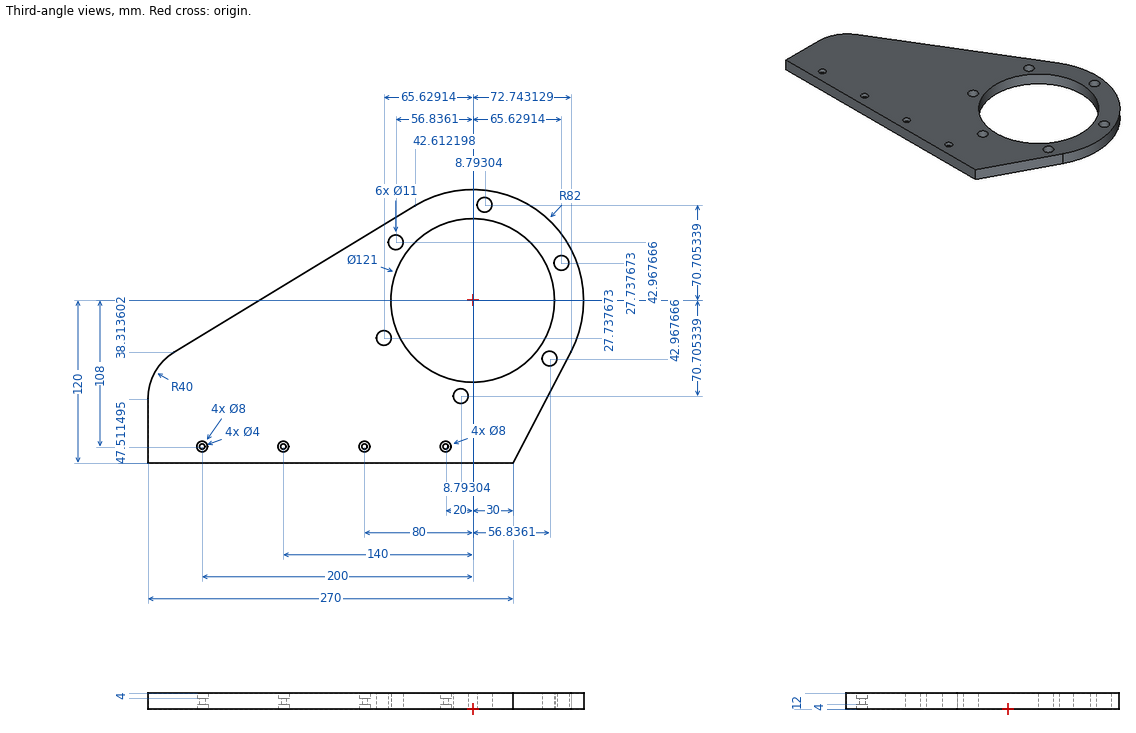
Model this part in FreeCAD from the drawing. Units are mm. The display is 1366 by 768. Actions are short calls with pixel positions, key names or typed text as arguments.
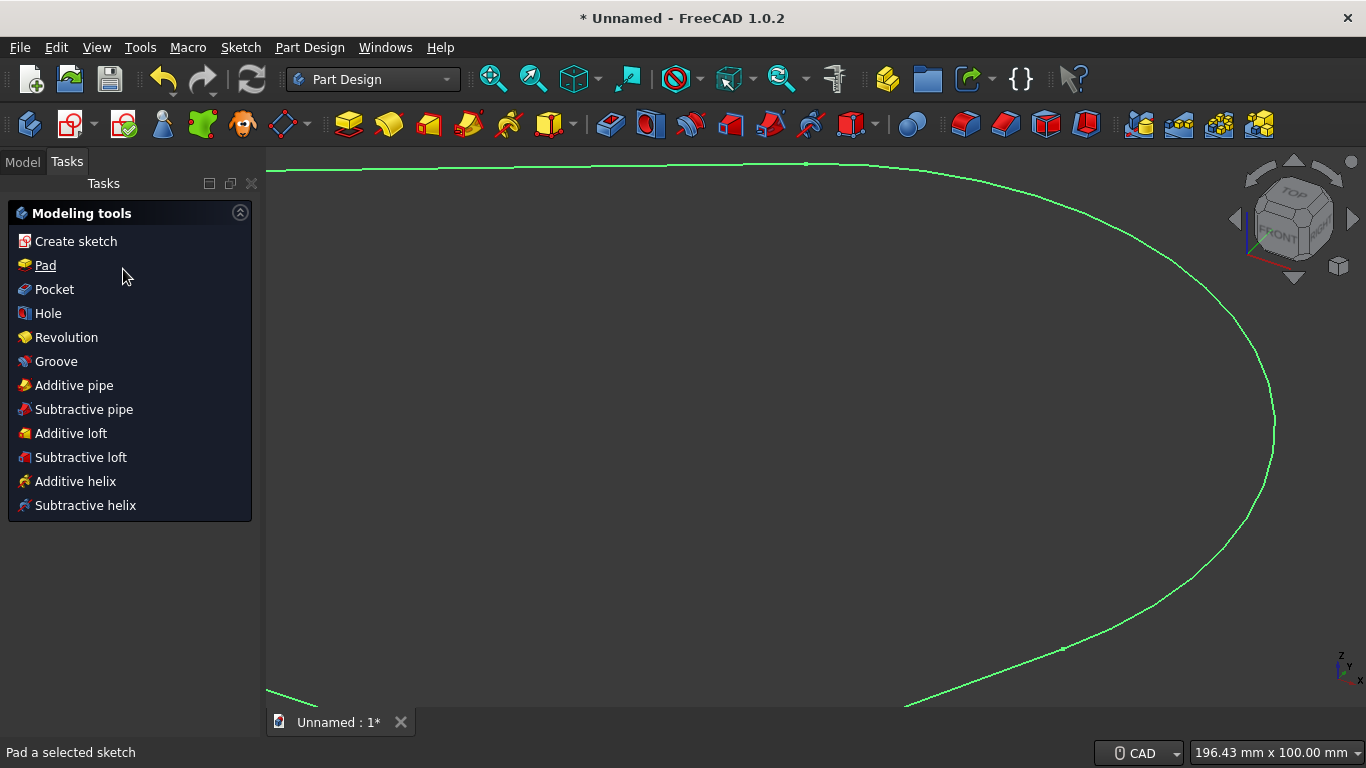
click(350, 124)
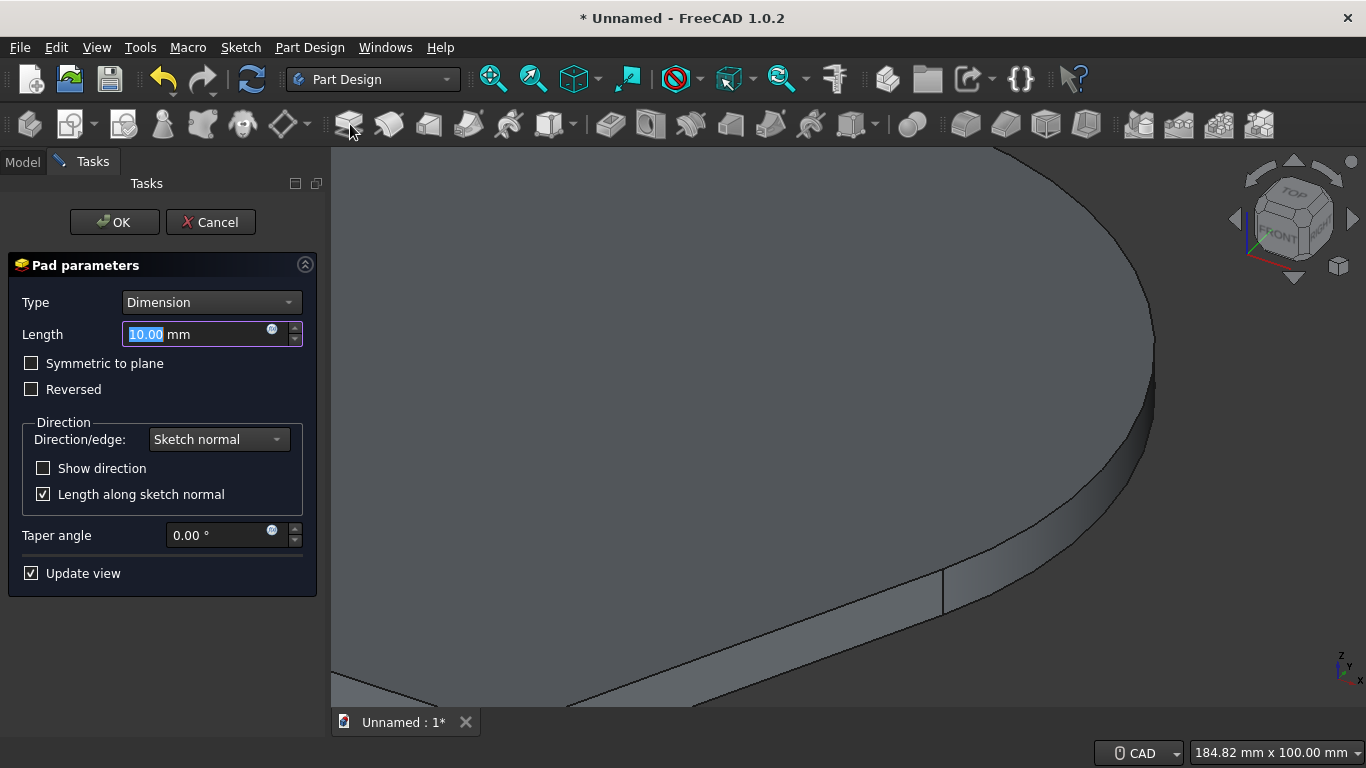
text(12)
key(Tab)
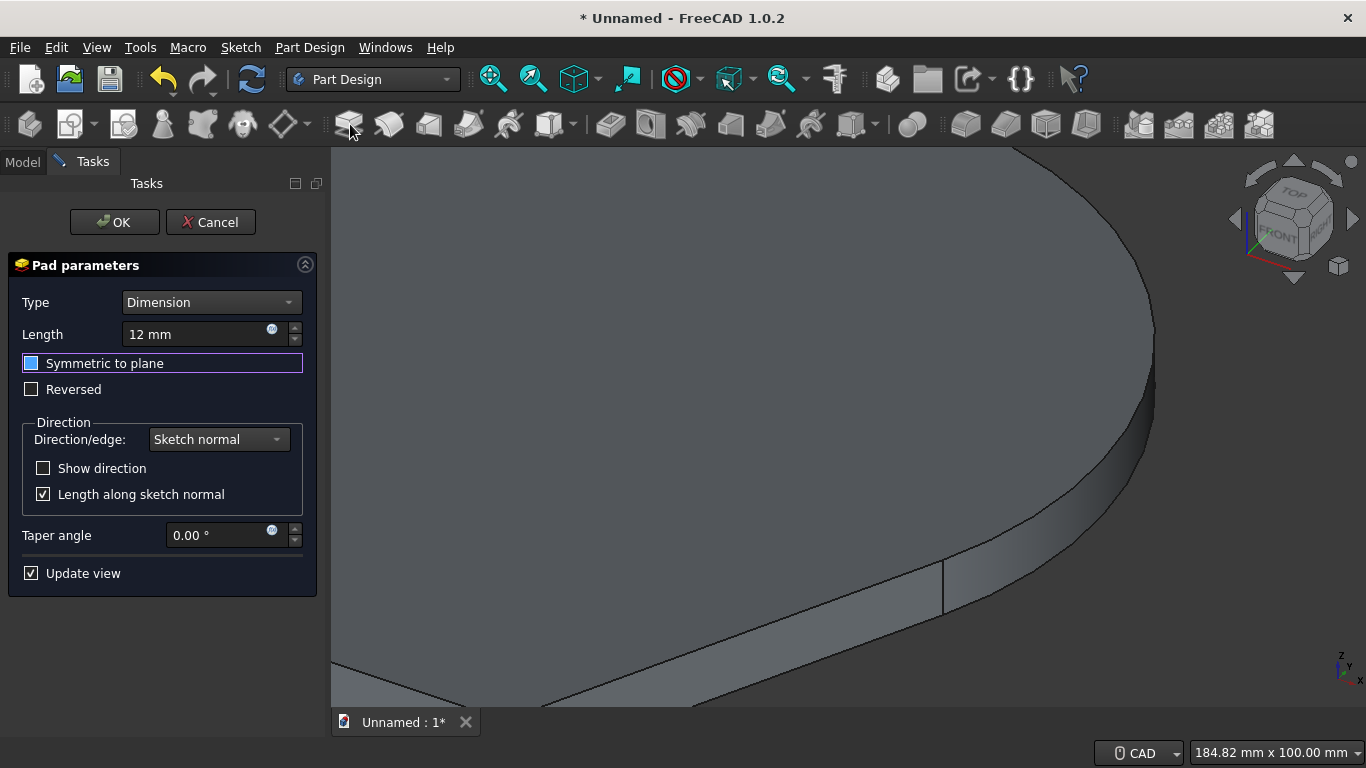
click(115, 222)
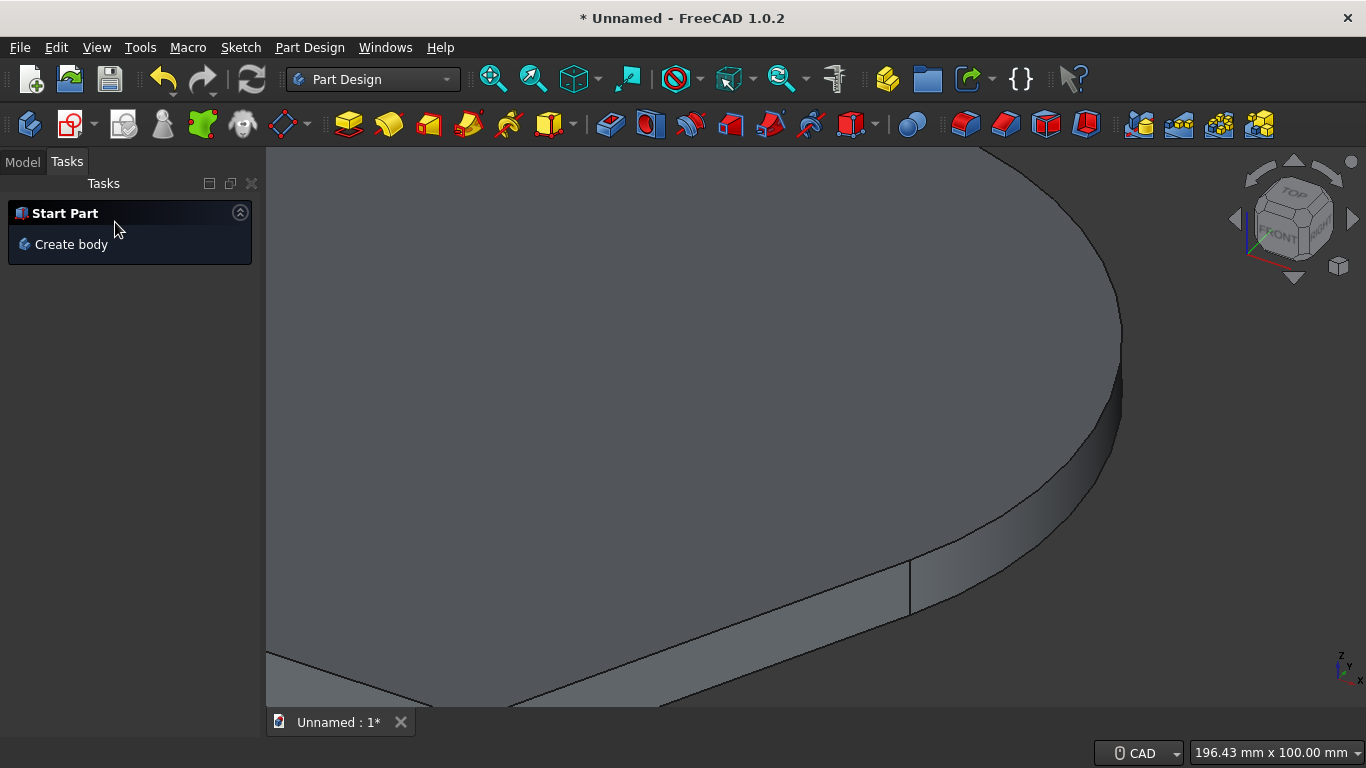
click(494, 80)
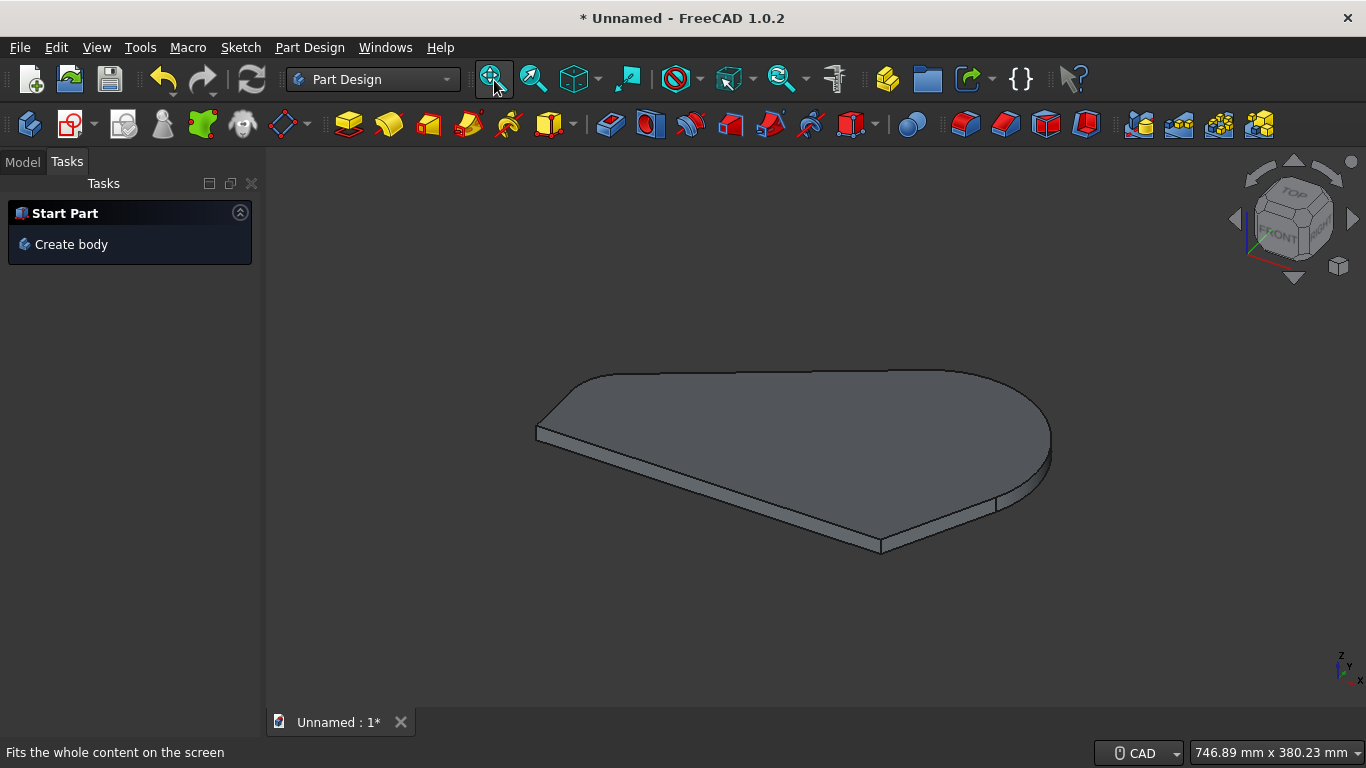
key(5)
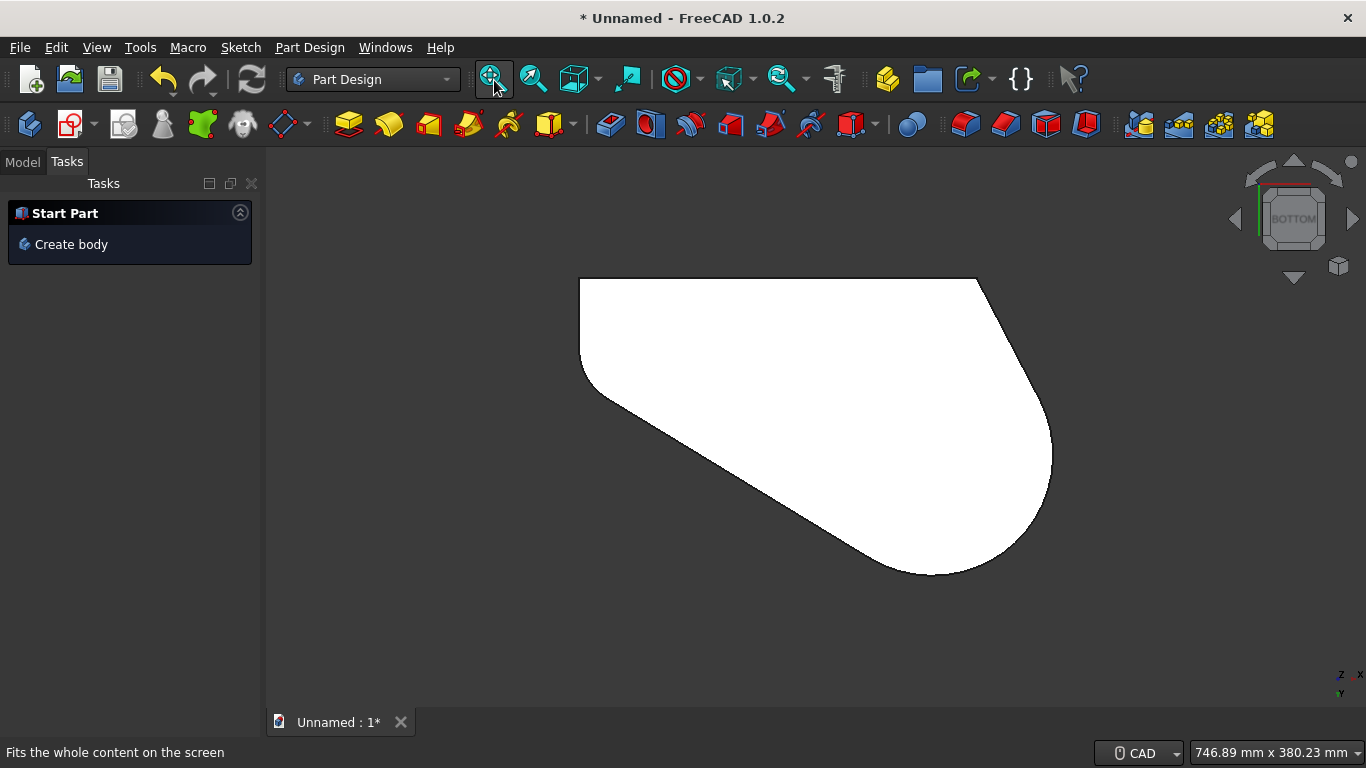
click(884, 426)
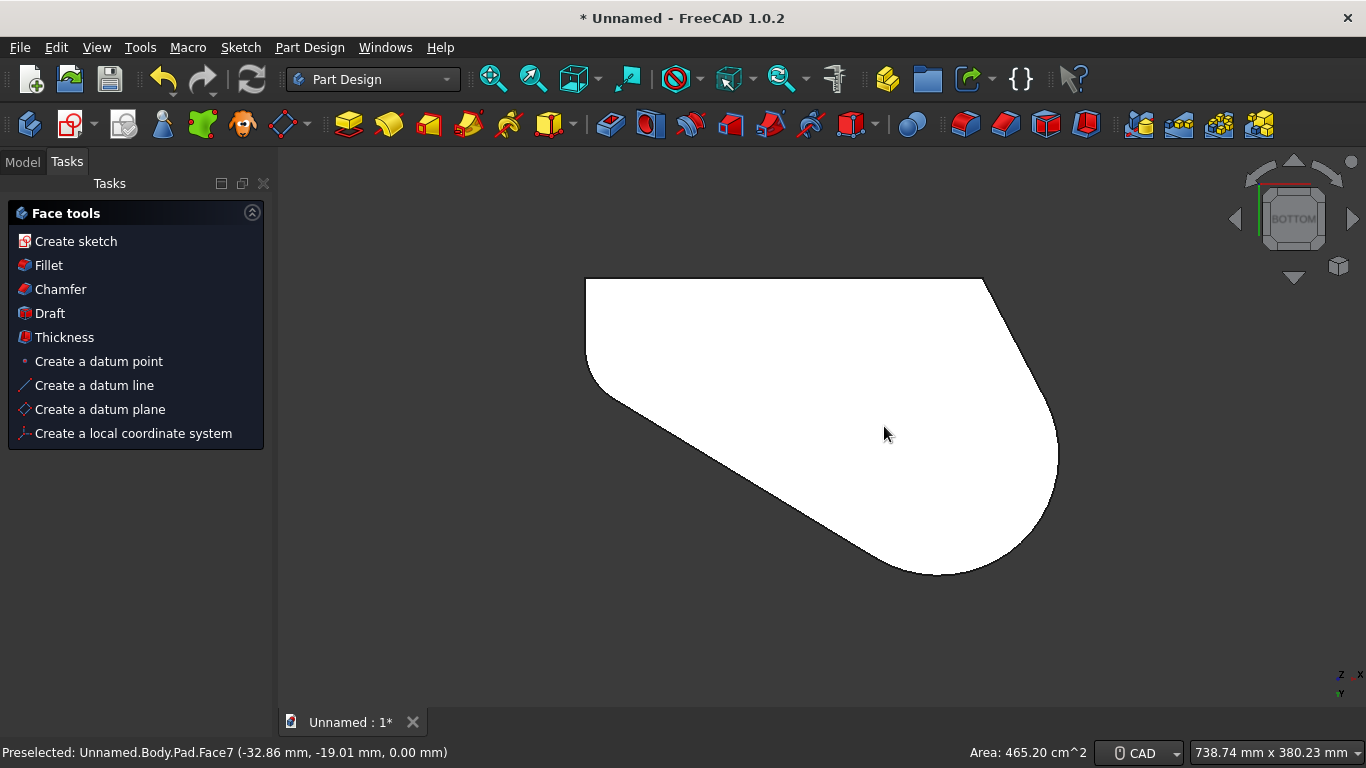
click(70, 124)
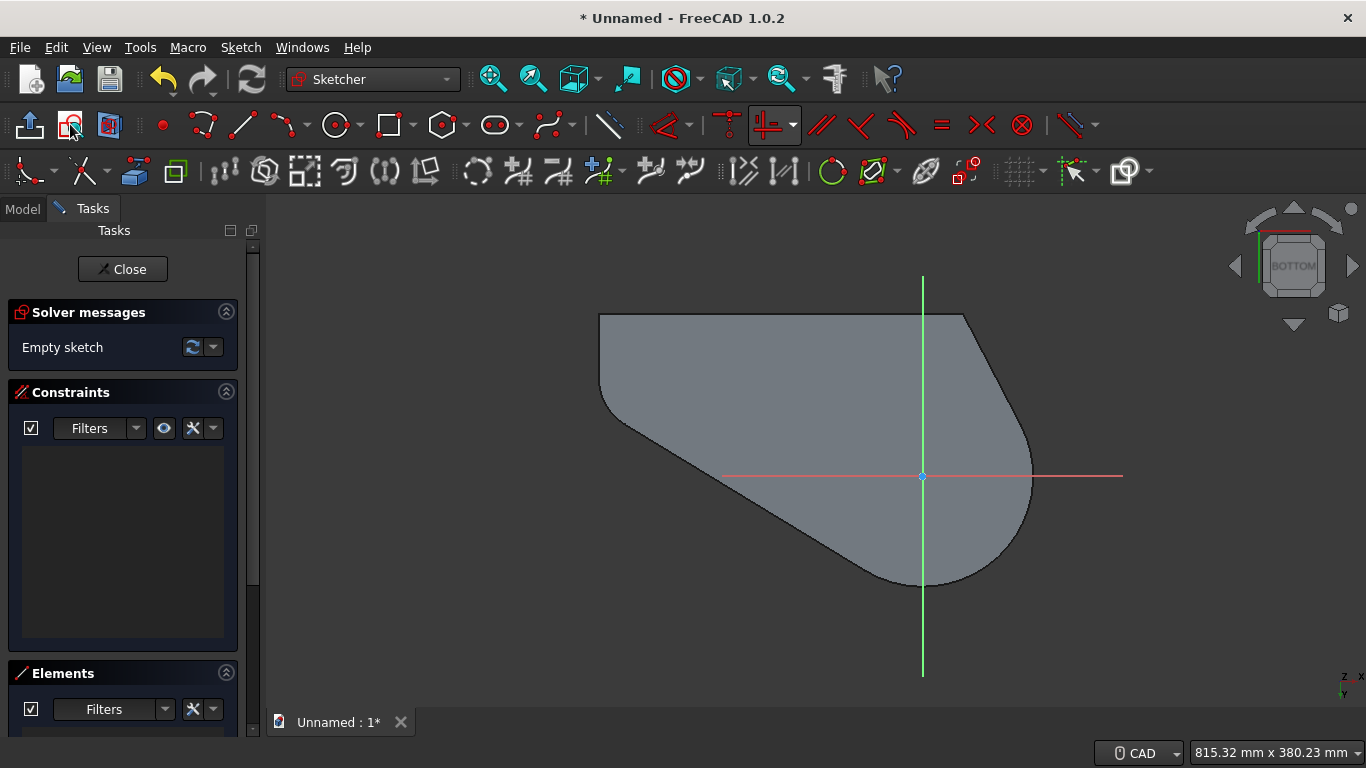
scroll(1136, 507, up, 3)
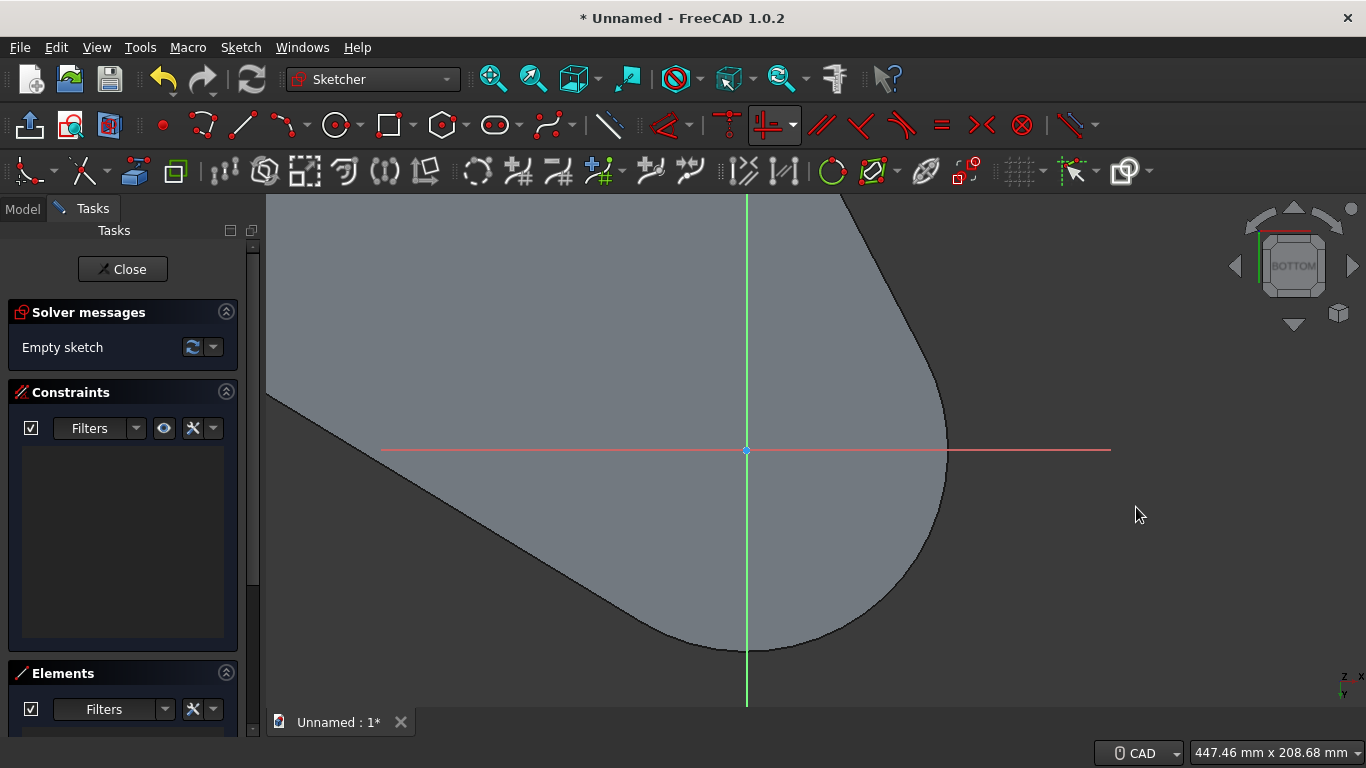
click(336, 126)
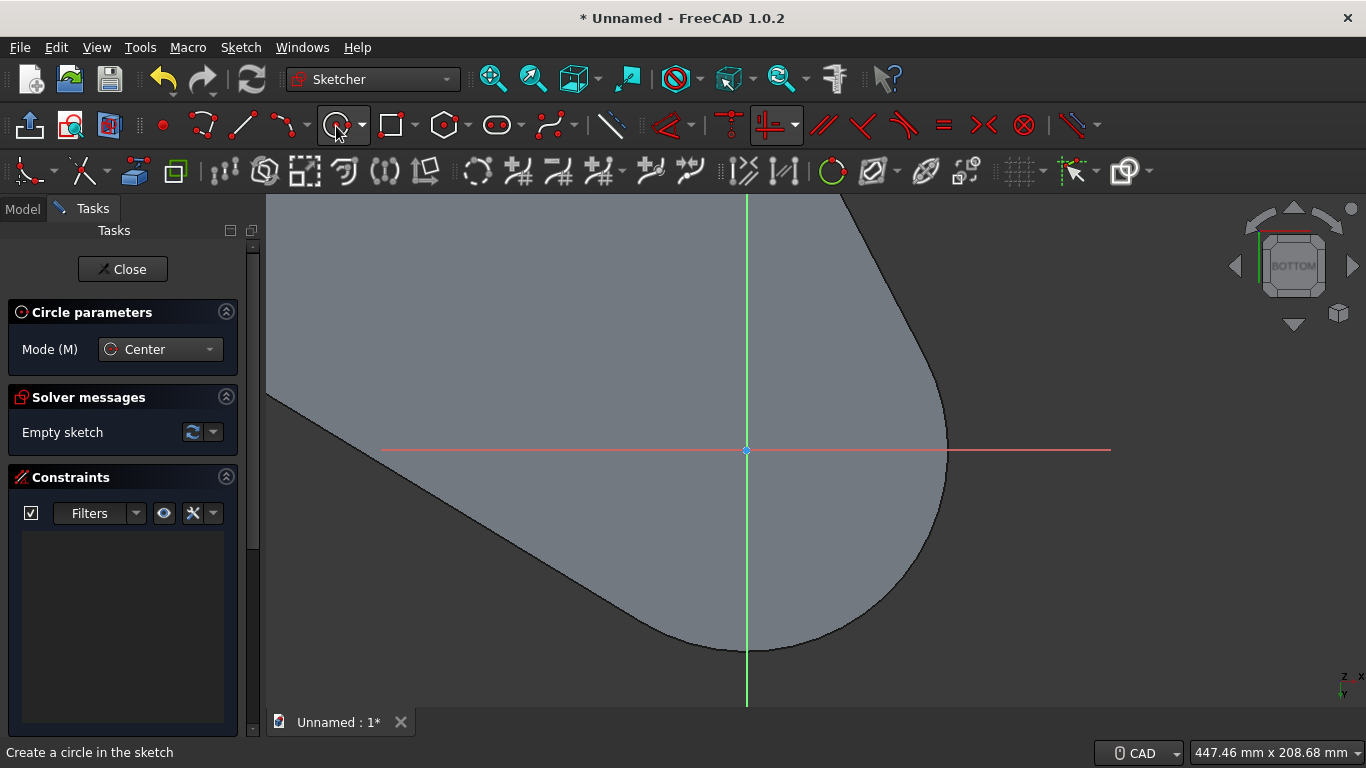
click(747, 450)
click(852, 345)
key(Escape)